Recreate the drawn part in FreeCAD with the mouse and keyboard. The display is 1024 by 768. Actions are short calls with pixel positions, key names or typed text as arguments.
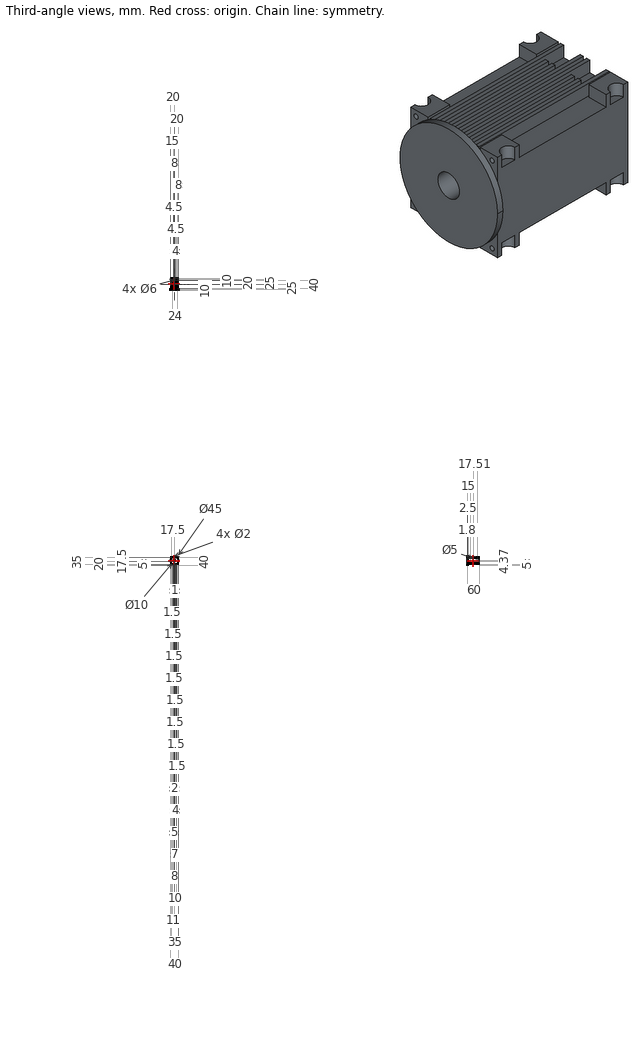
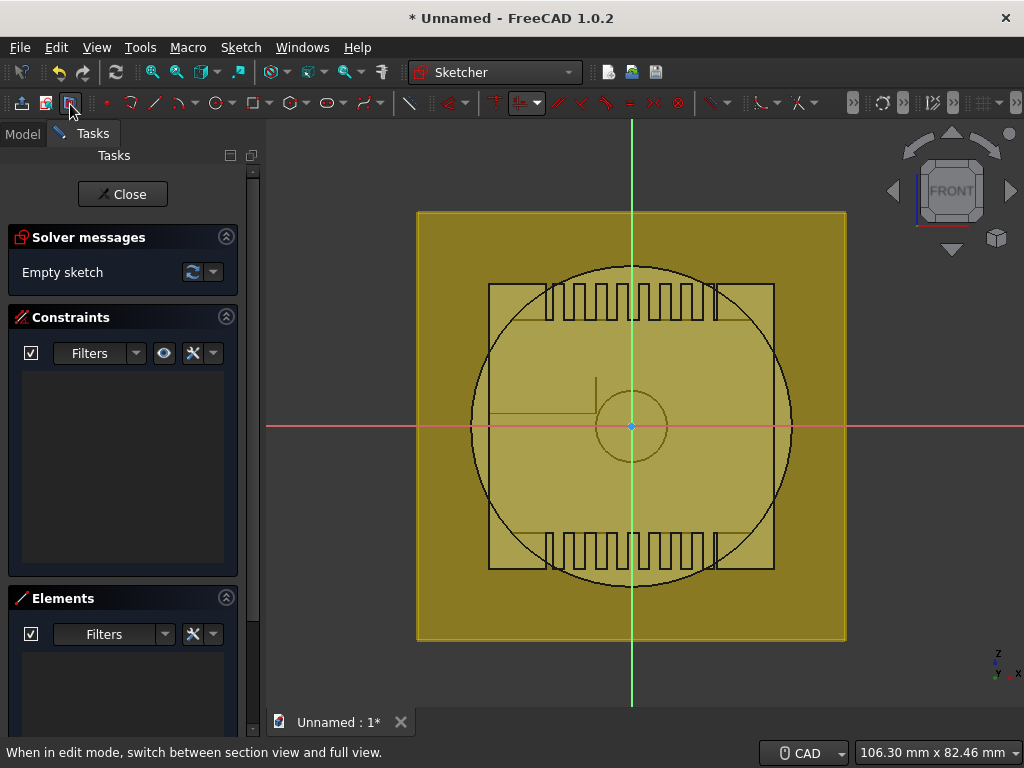
scroll(743, 454, up, 2)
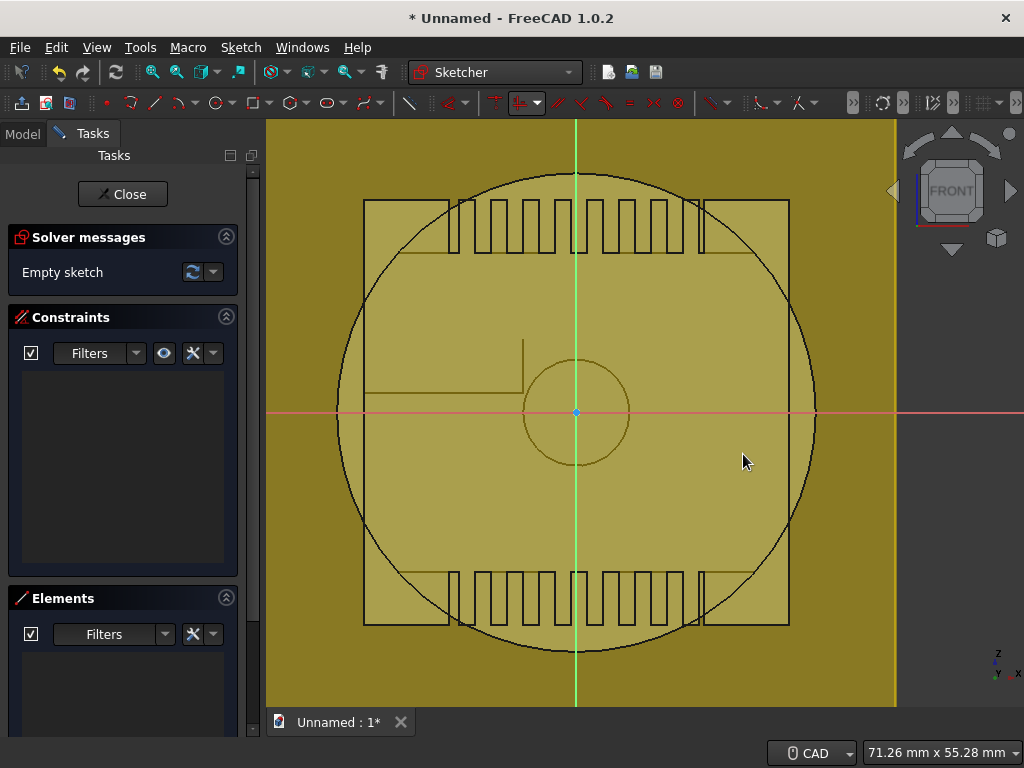
key(g)
key(c)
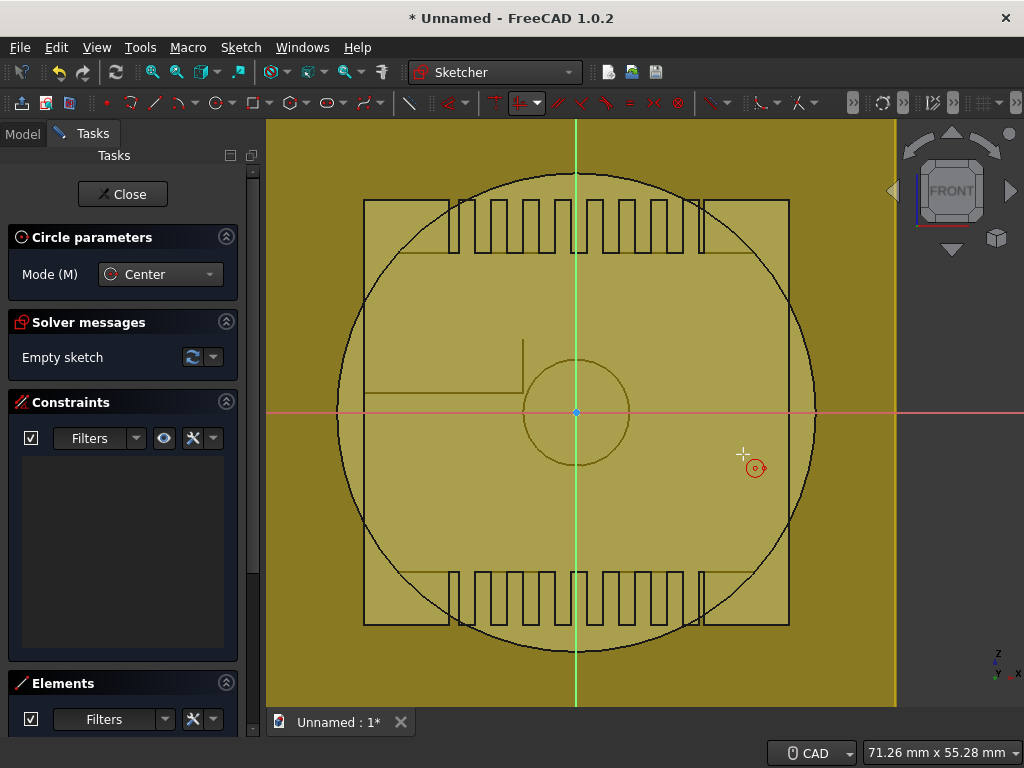
scroll(390, 227, up, 4)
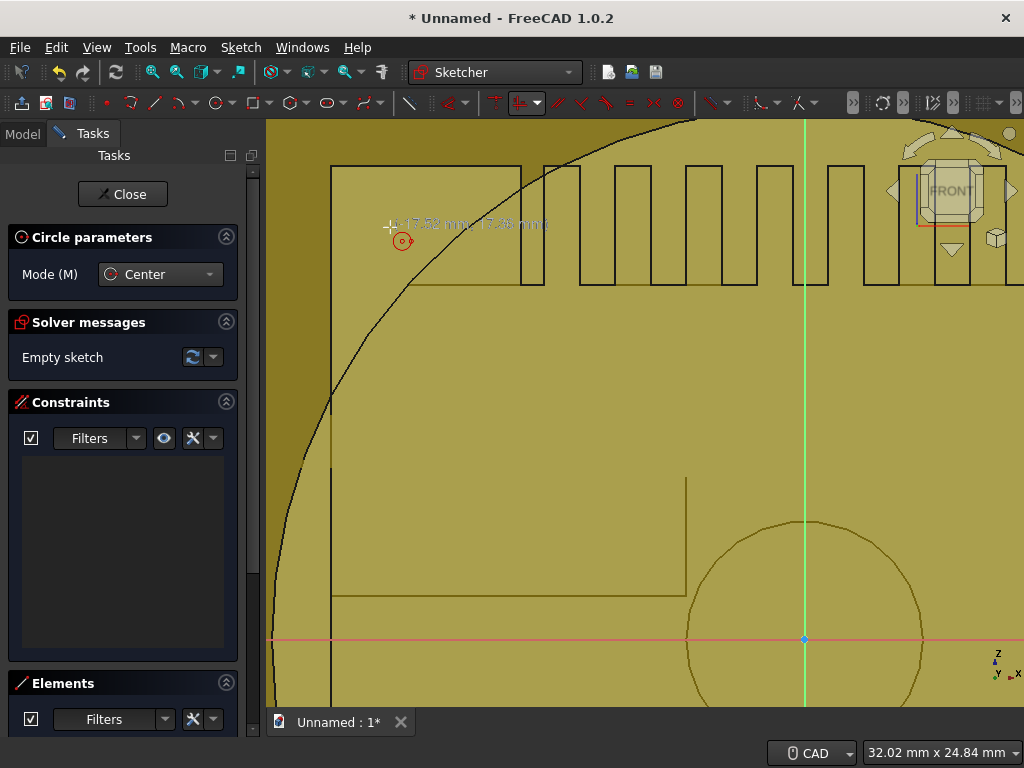
click(390, 226)
click(407, 209)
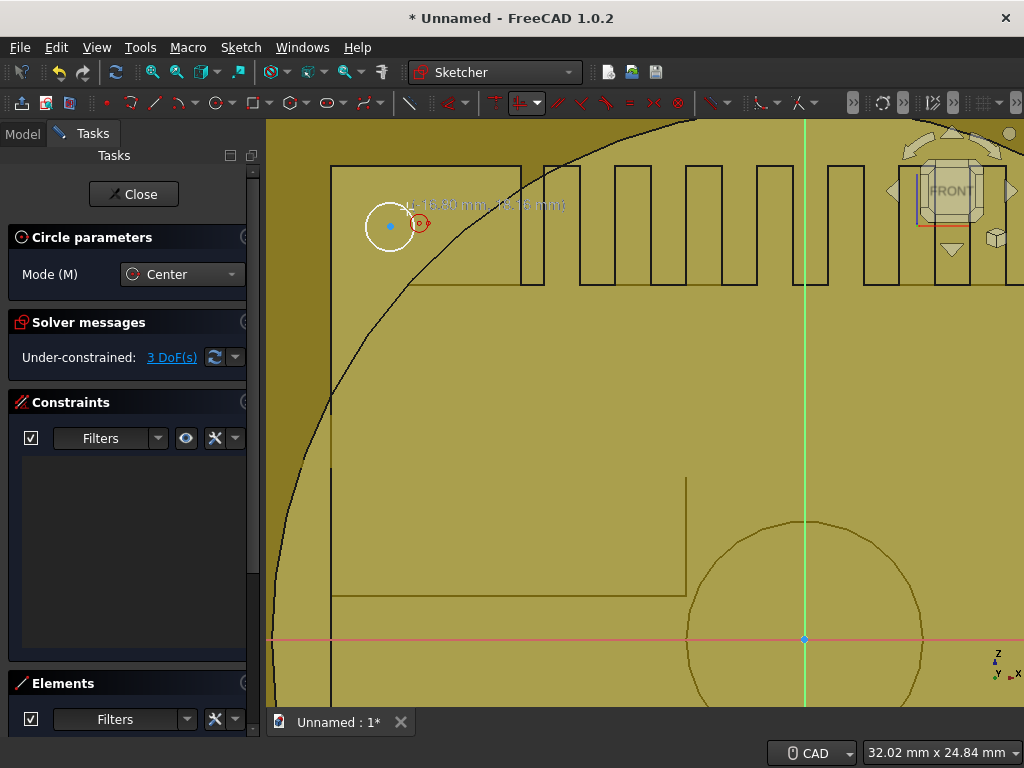
scroll(390, 228, down, 4)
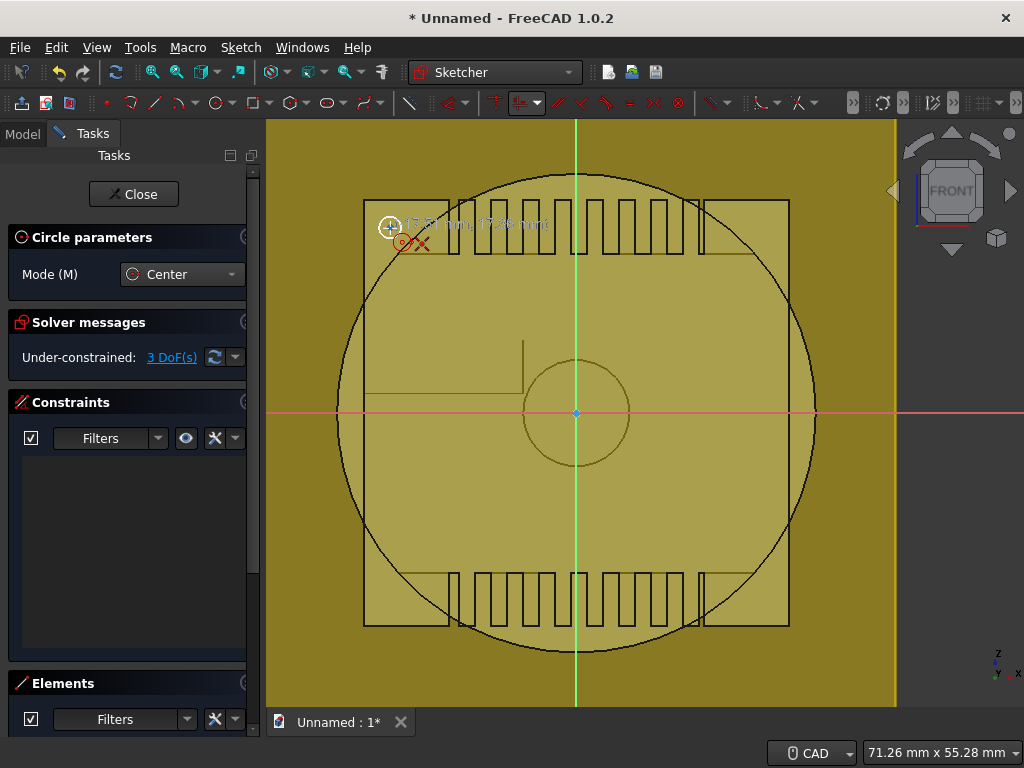
scroll(390, 599, up, 4)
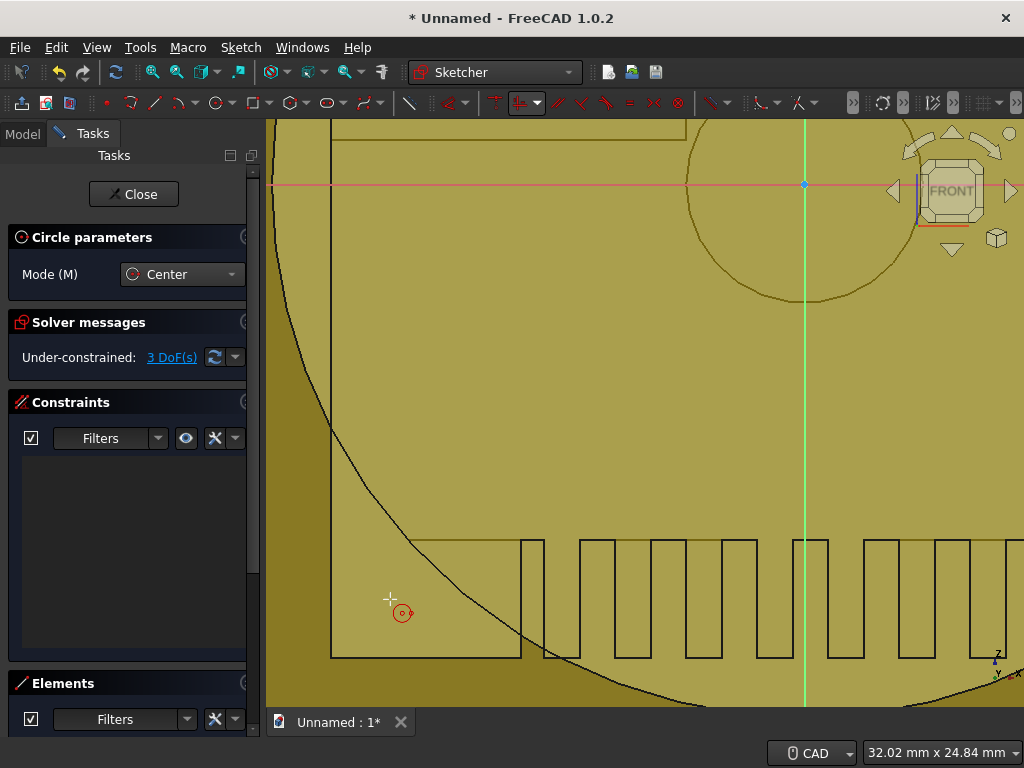
click(390, 599)
click(407, 582)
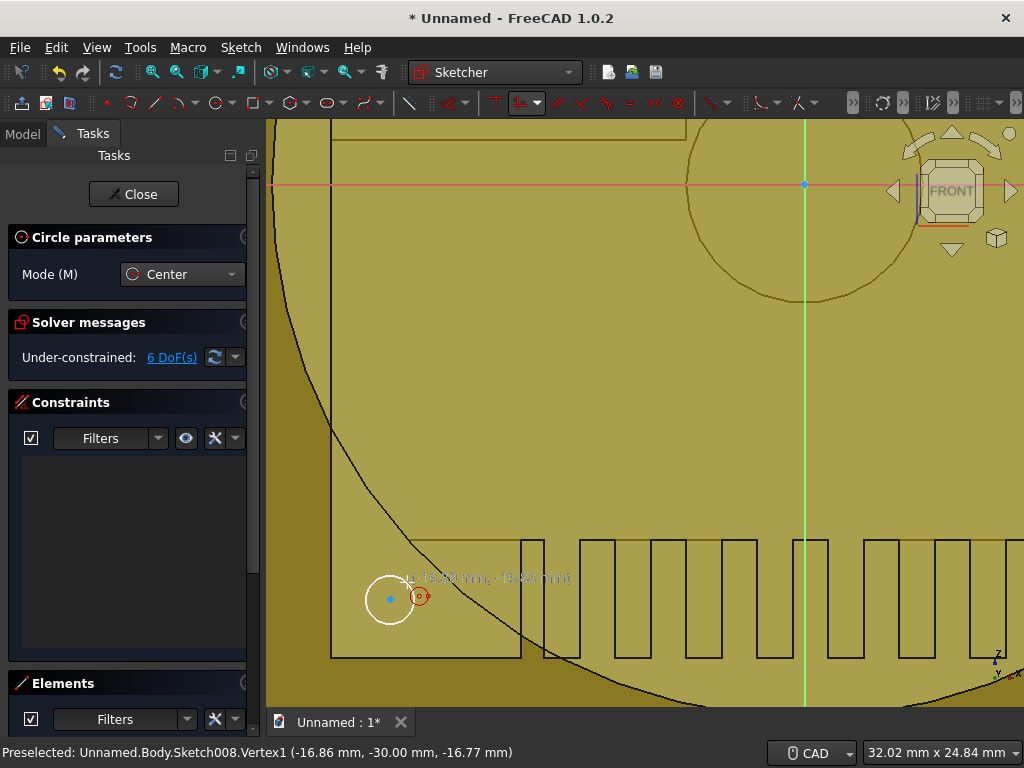
scroll(390, 599, down, 4)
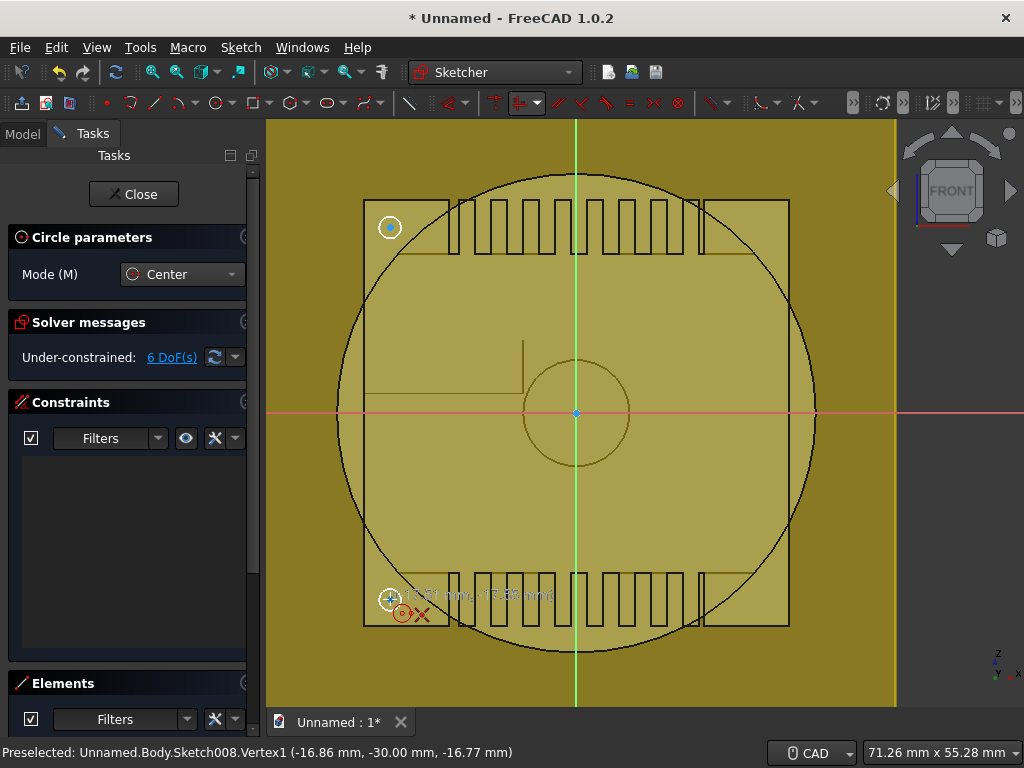
scroll(763, 599, up, 4)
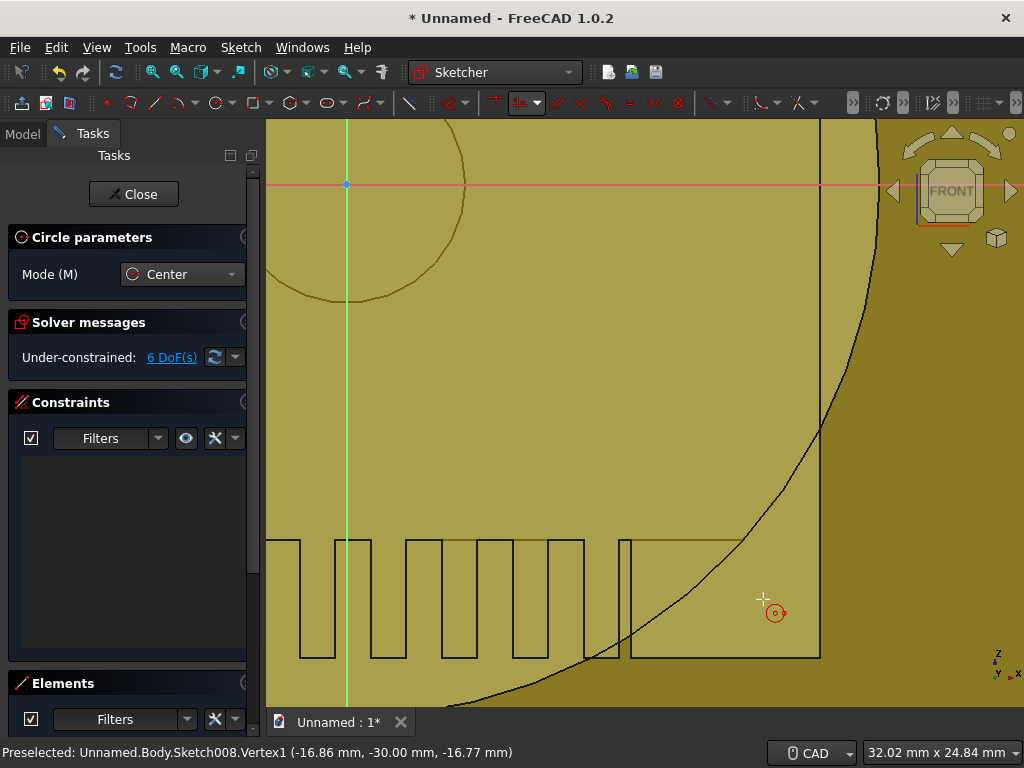
click(761, 599)
click(778, 582)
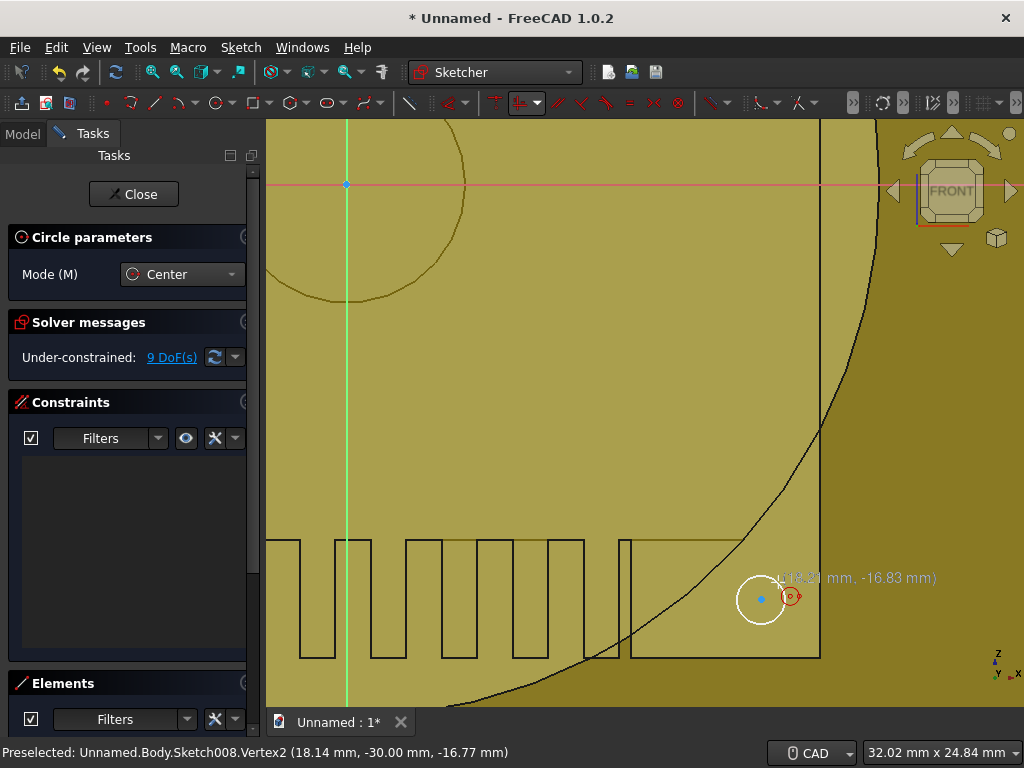
scroll(764, 599, down, 4)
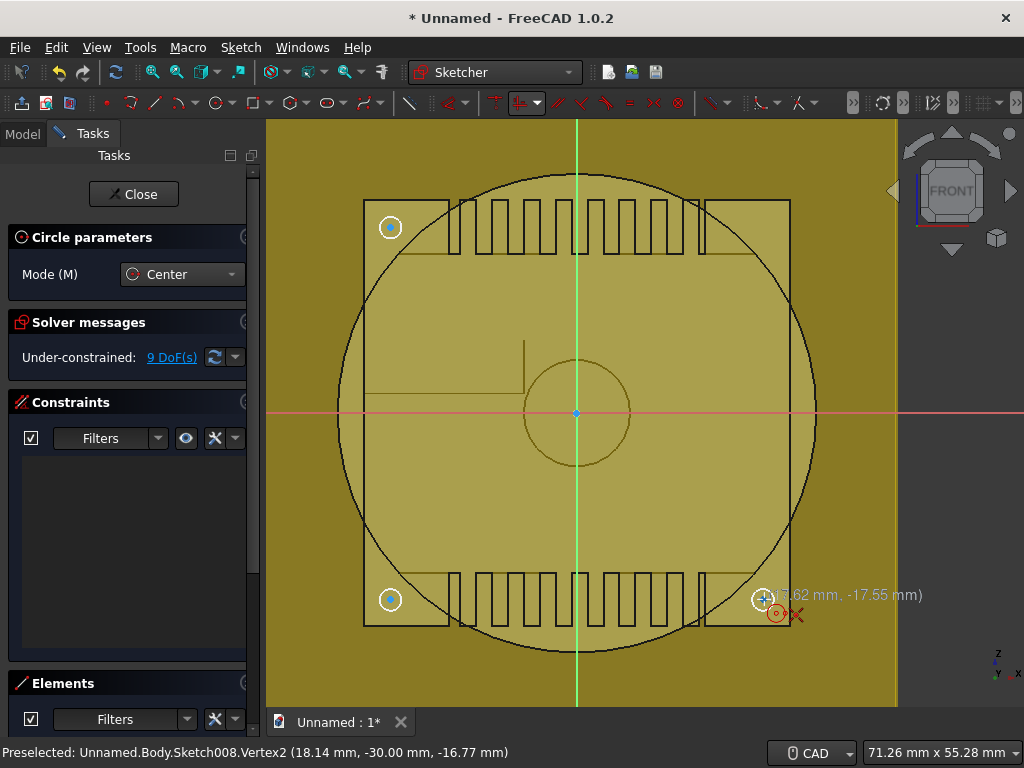
scroll(763, 227, up, 4)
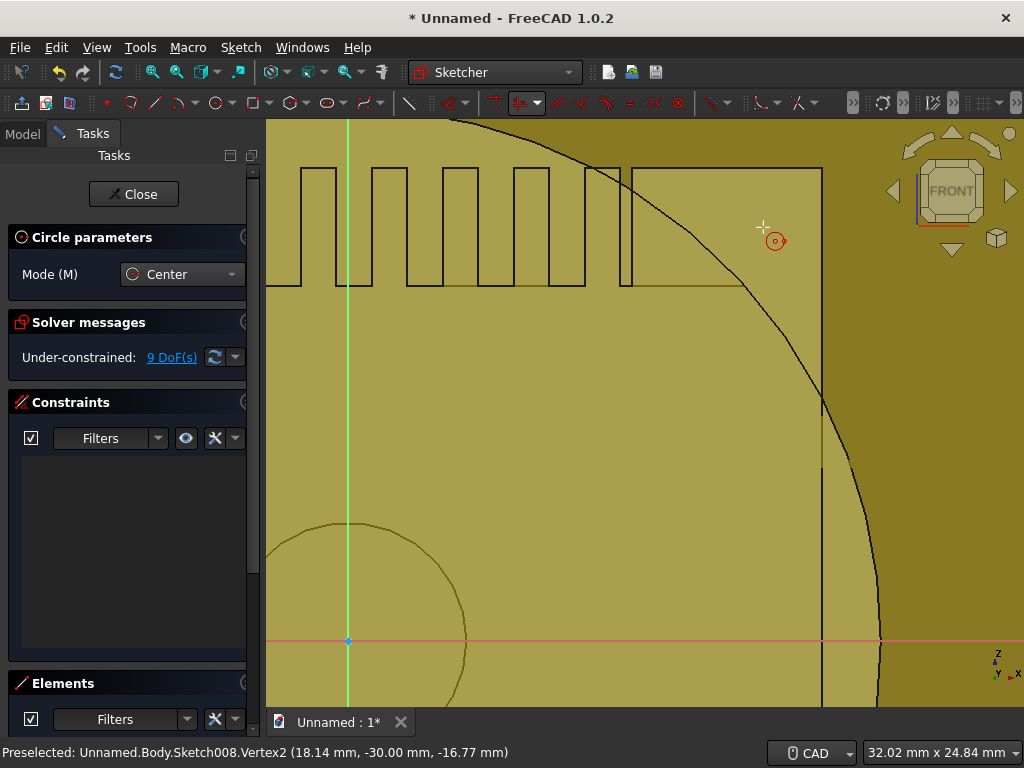
click(762, 227)
click(779, 210)
key(Escape)